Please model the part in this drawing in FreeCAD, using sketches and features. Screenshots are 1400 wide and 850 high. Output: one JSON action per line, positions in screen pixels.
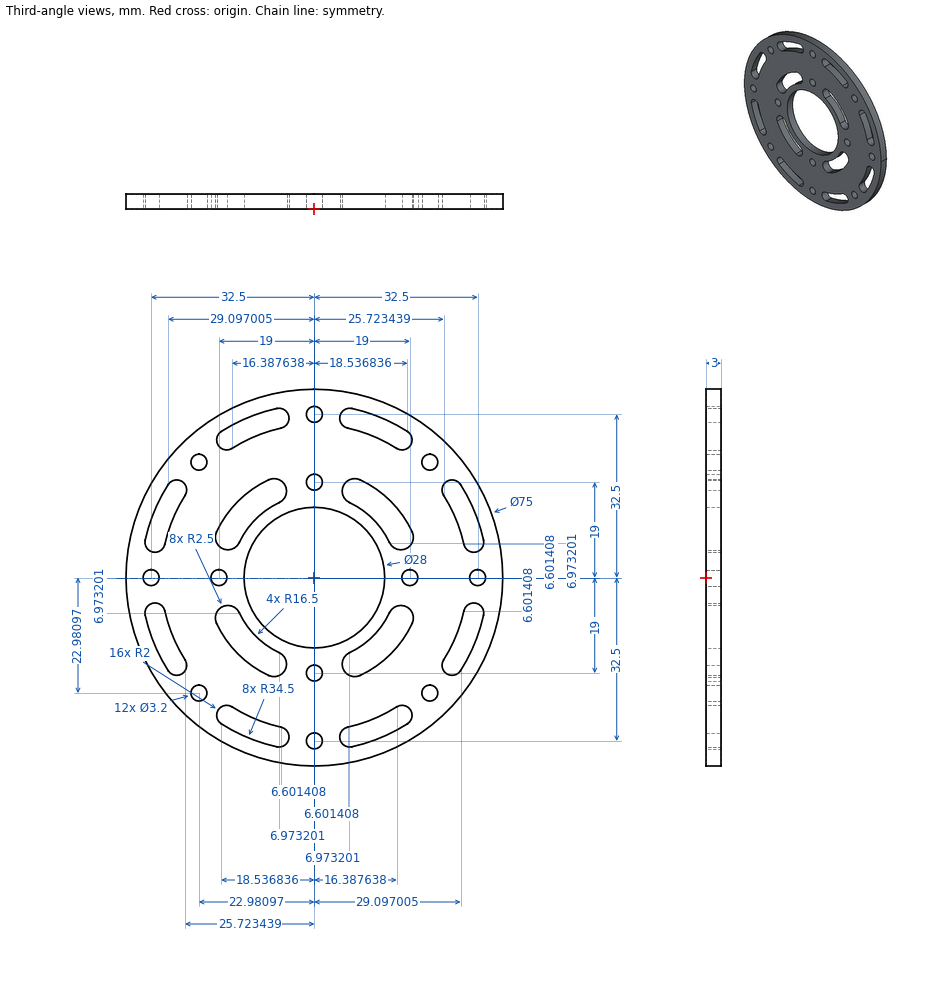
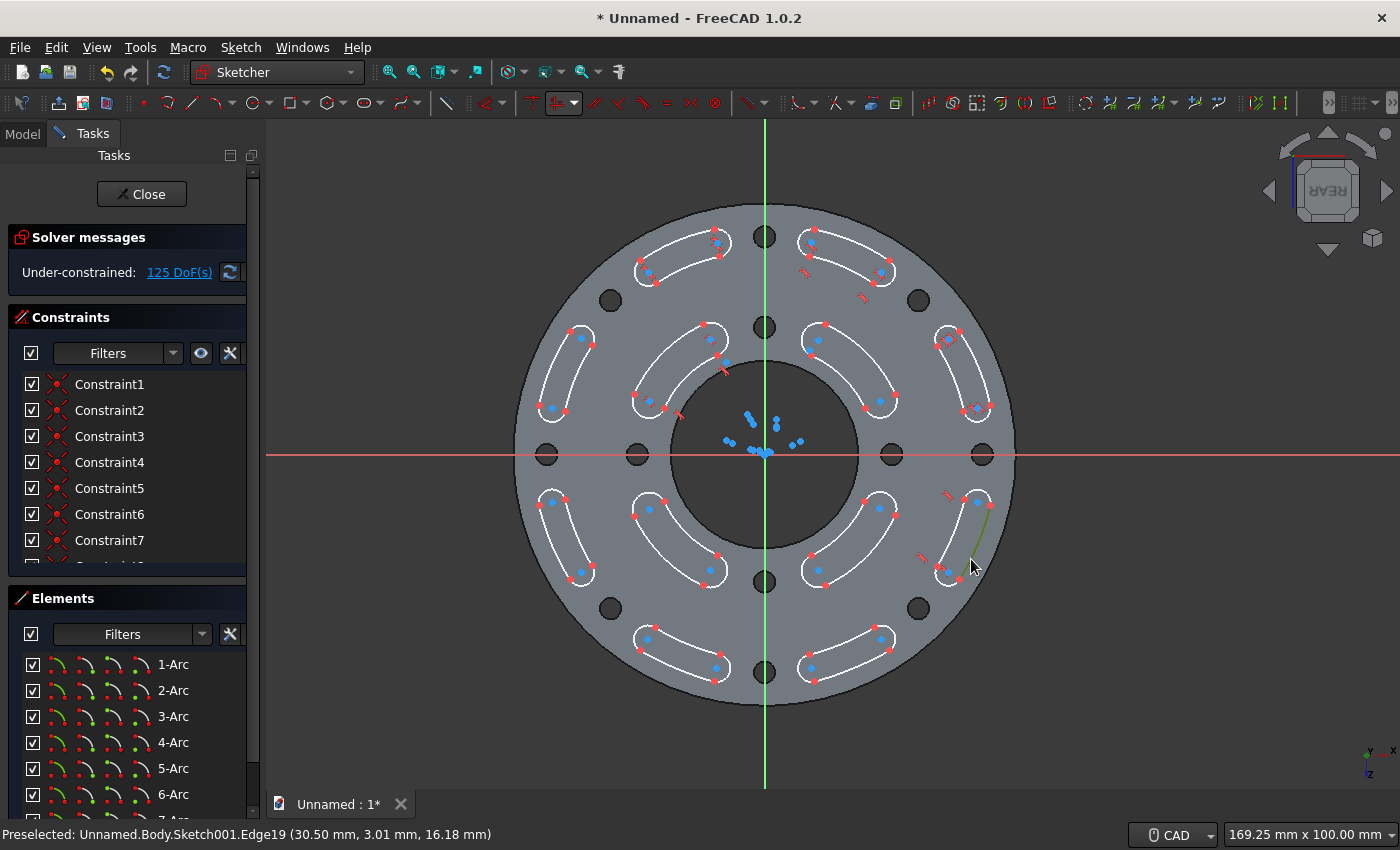
{"action": "left_click", "coordinate": [987, 494]}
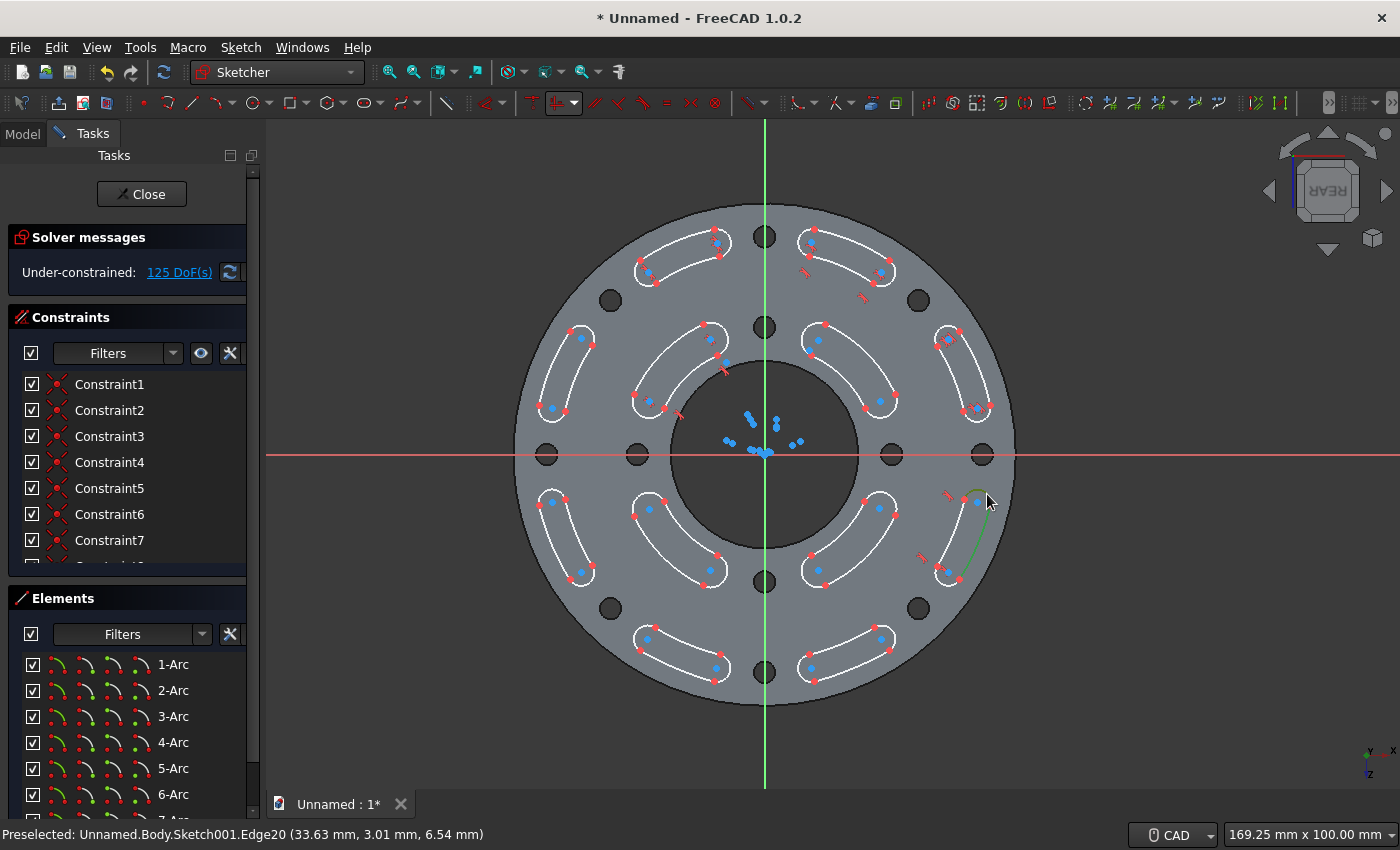
{"action": "left_click", "coordinate": [644, 104]}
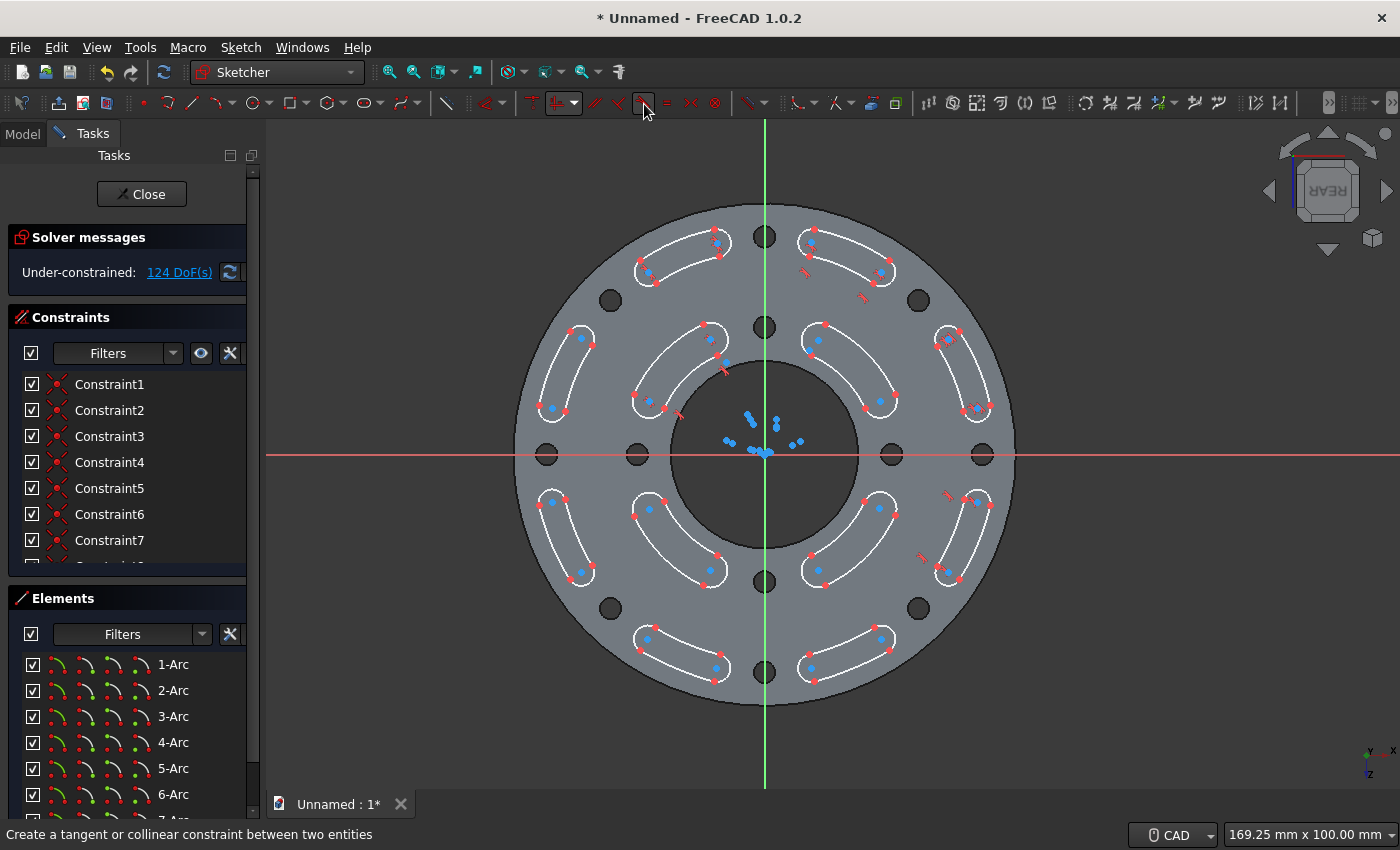
{"action": "left_click", "coordinate": [799, 662]}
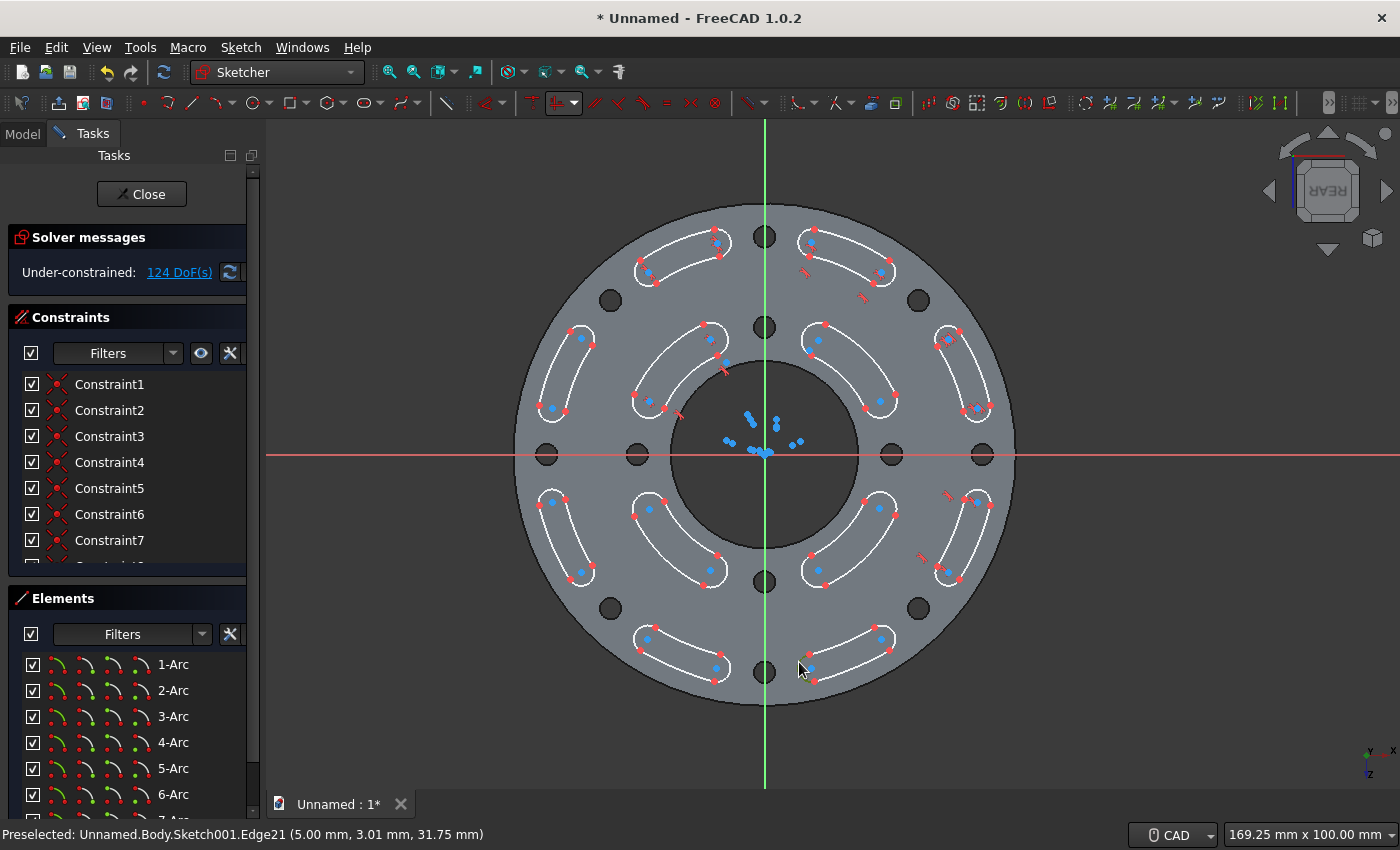
{"action": "left_click", "coordinate": [838, 674]}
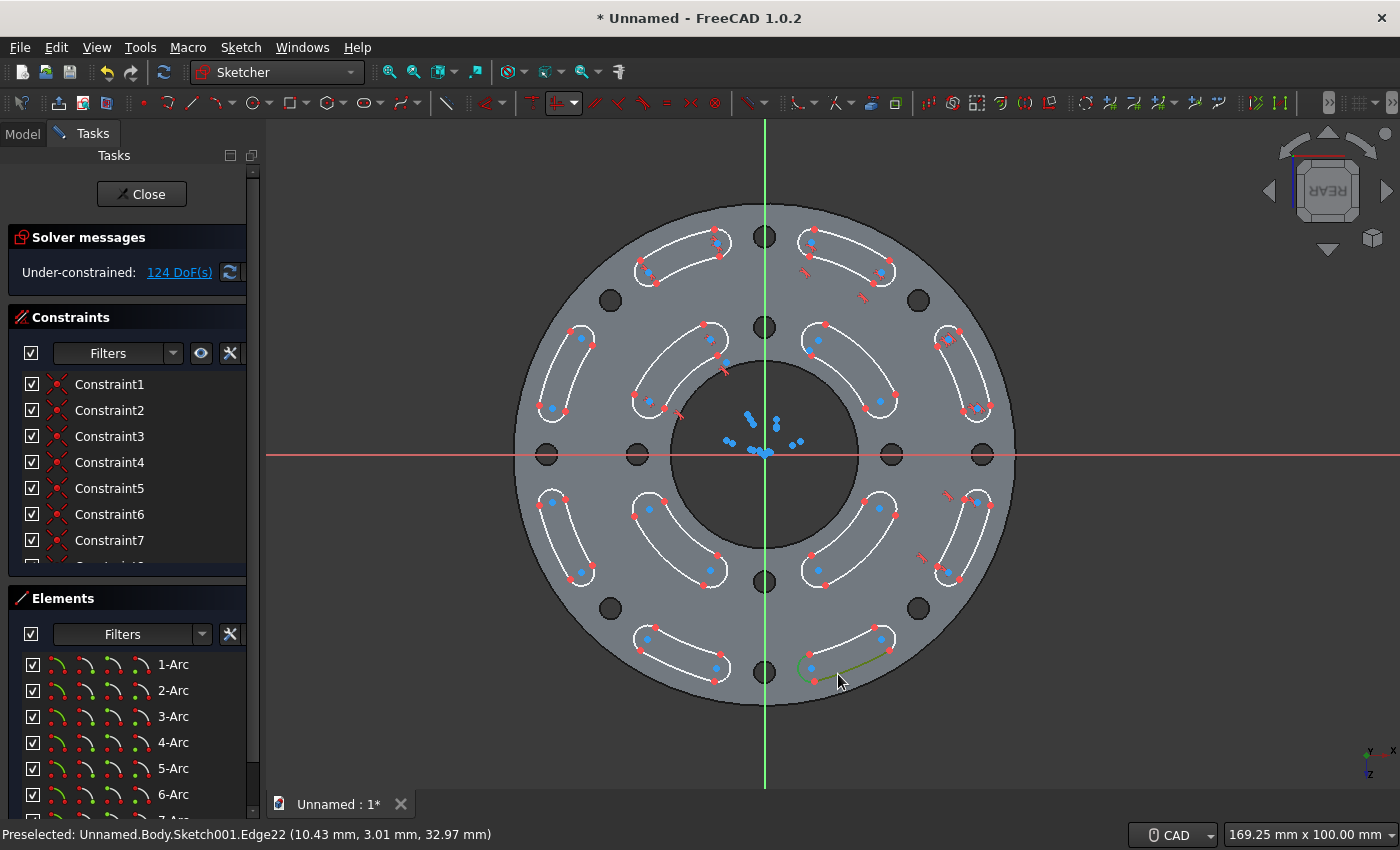
{"action": "left_click", "coordinate": [644, 104]}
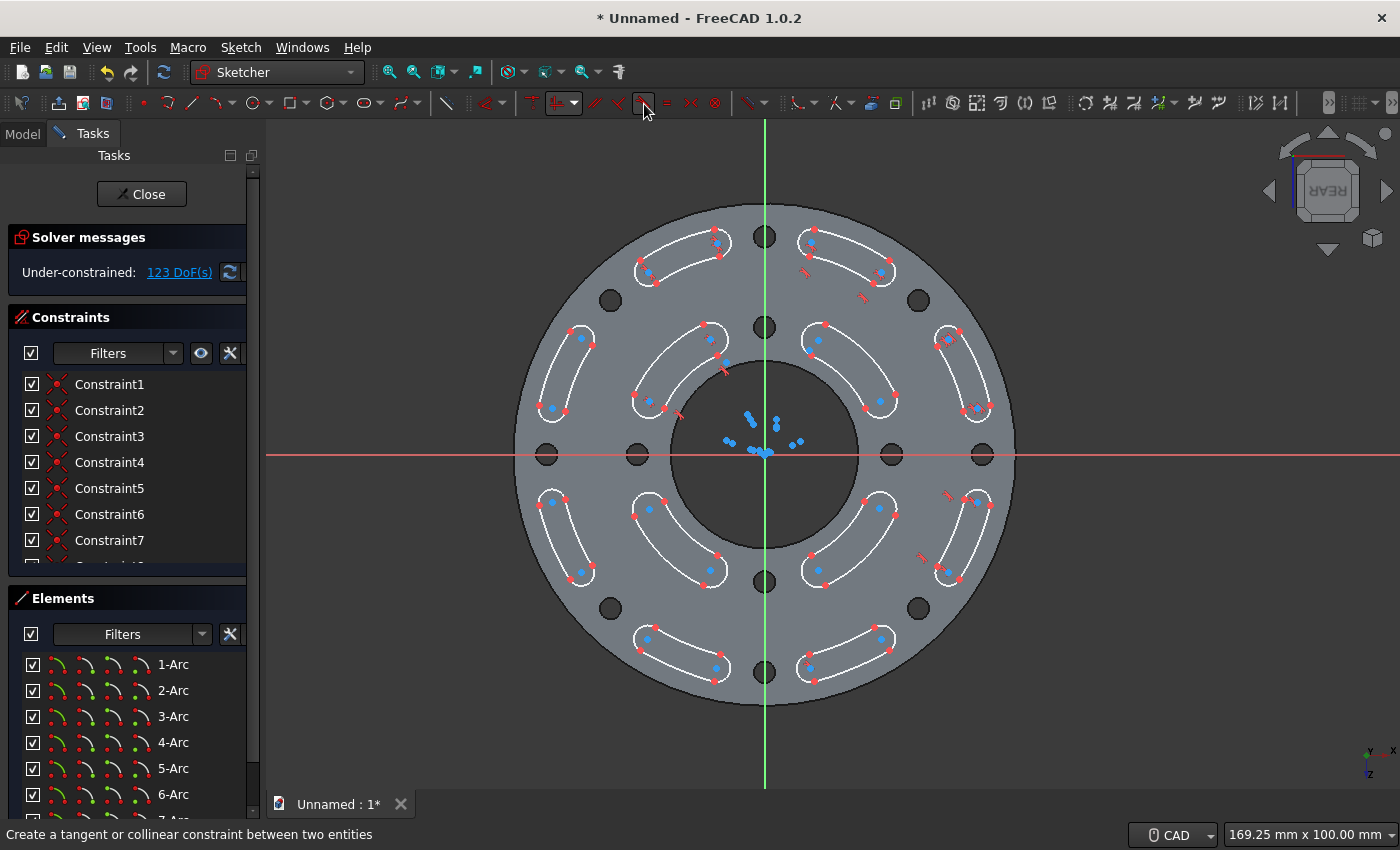
{"action": "left_click", "coordinate": [798, 662]}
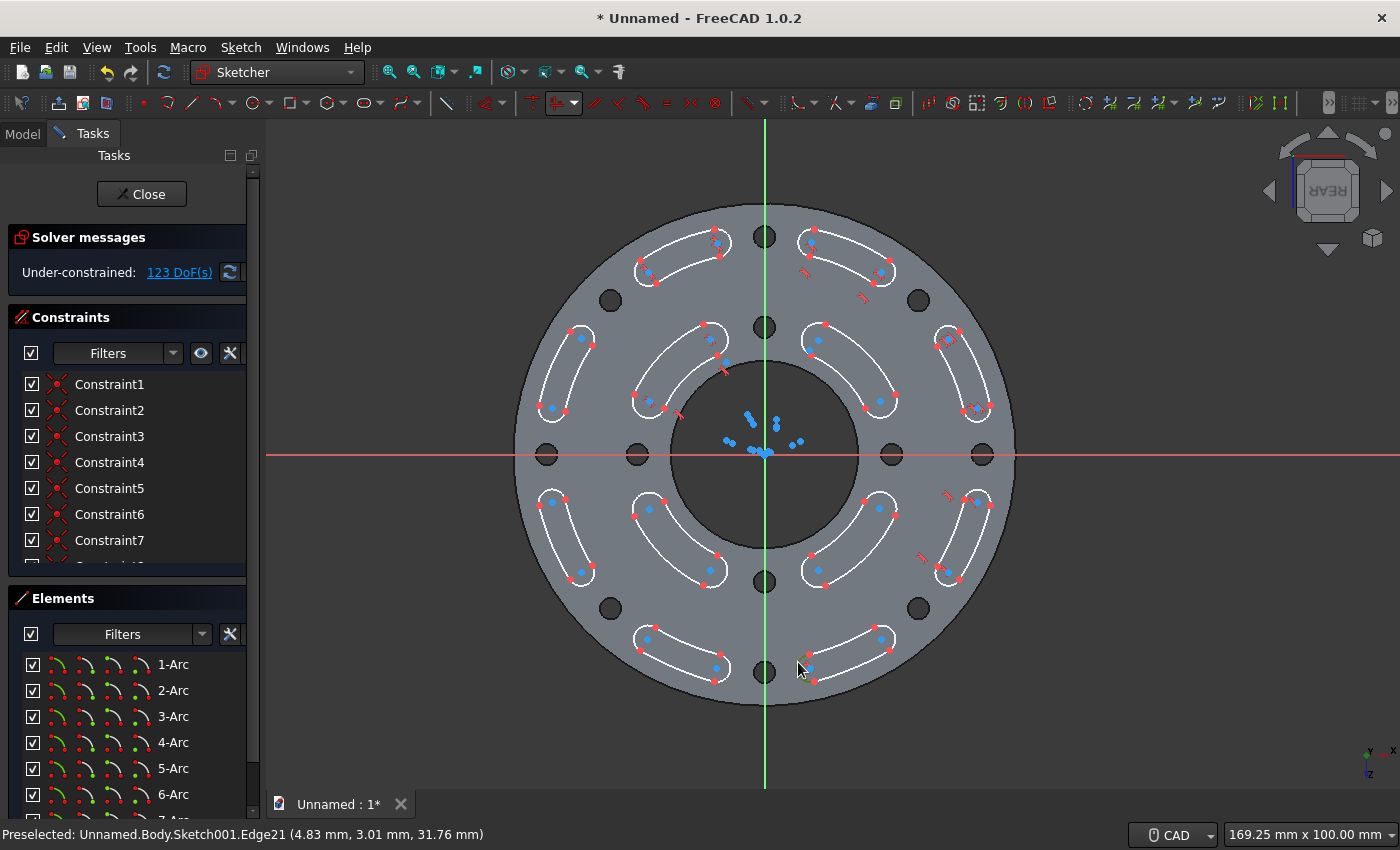
{"action": "left_click", "coordinate": [830, 649]}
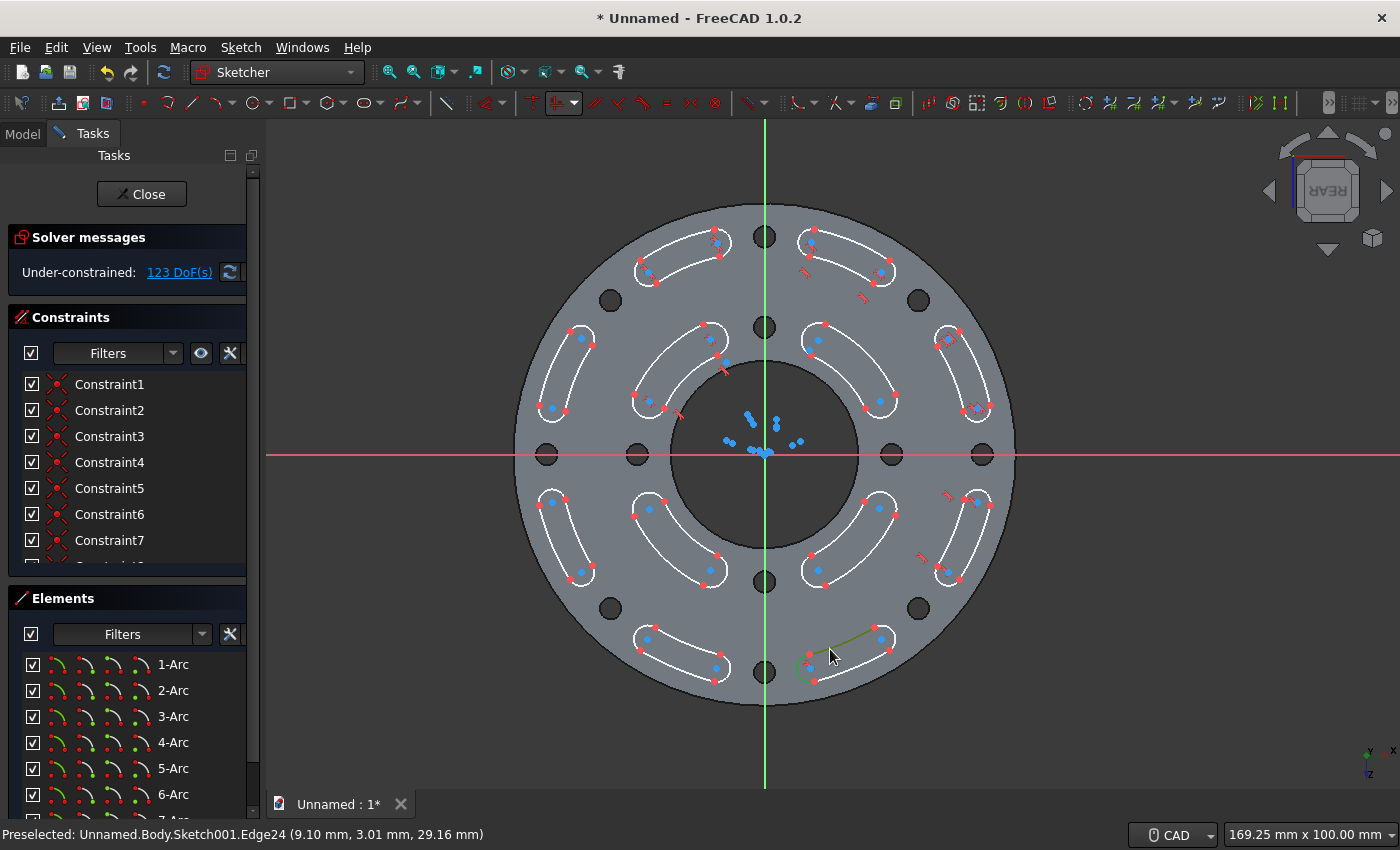
{"action": "left_click", "coordinate": [644, 104]}